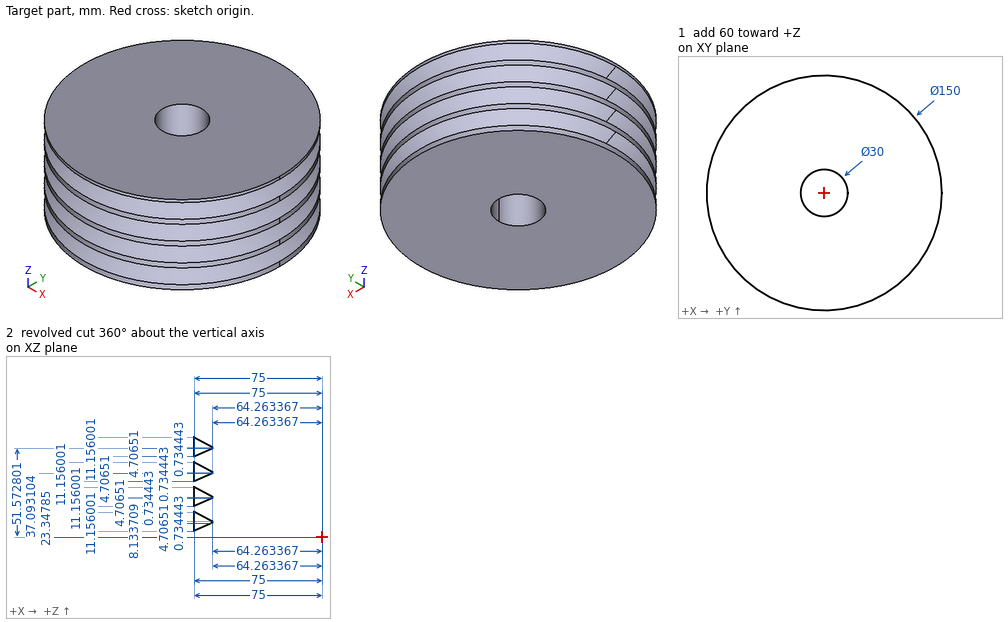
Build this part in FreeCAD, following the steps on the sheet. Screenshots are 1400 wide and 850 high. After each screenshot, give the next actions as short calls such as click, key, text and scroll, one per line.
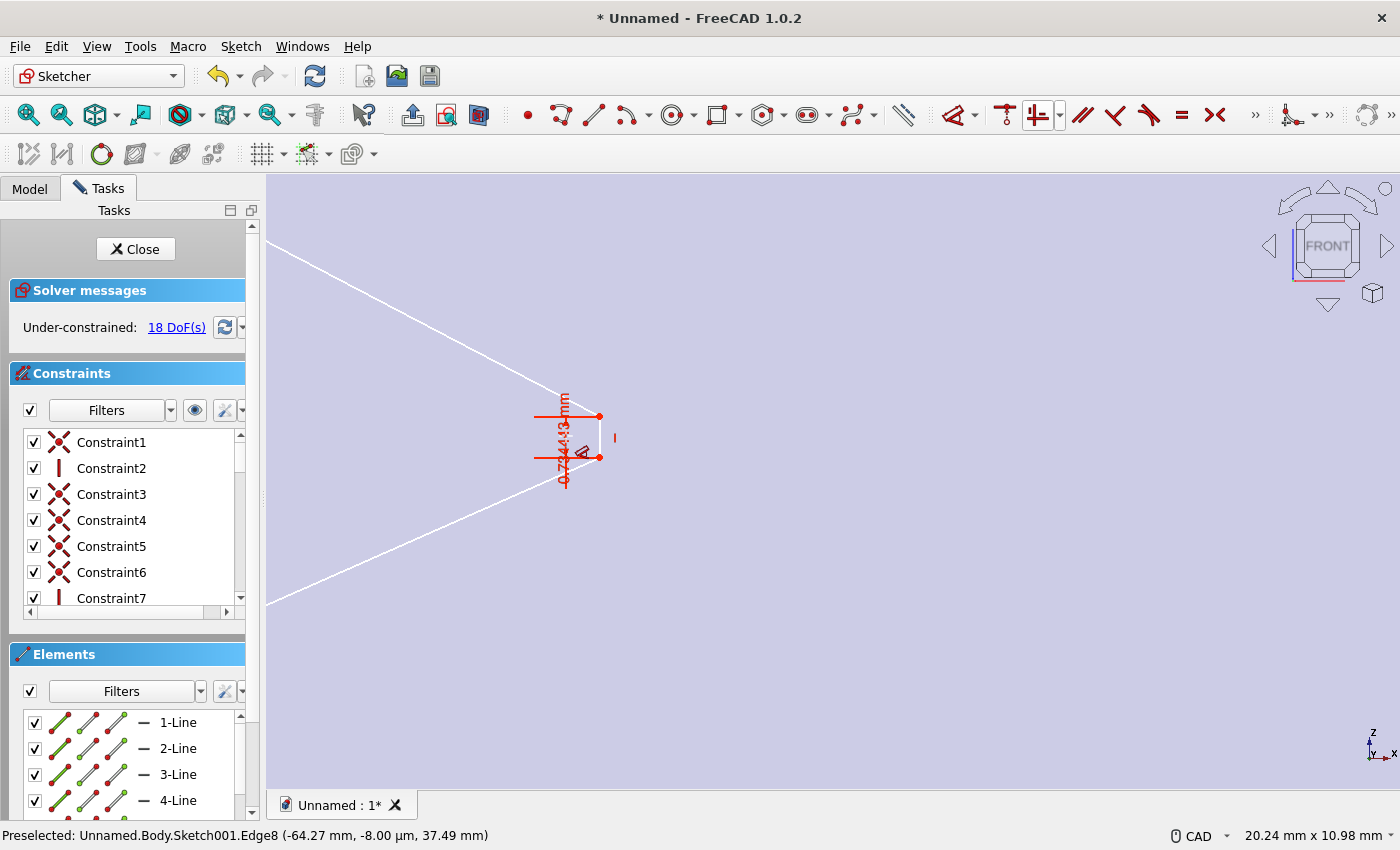
scroll(598, 429, down, 11)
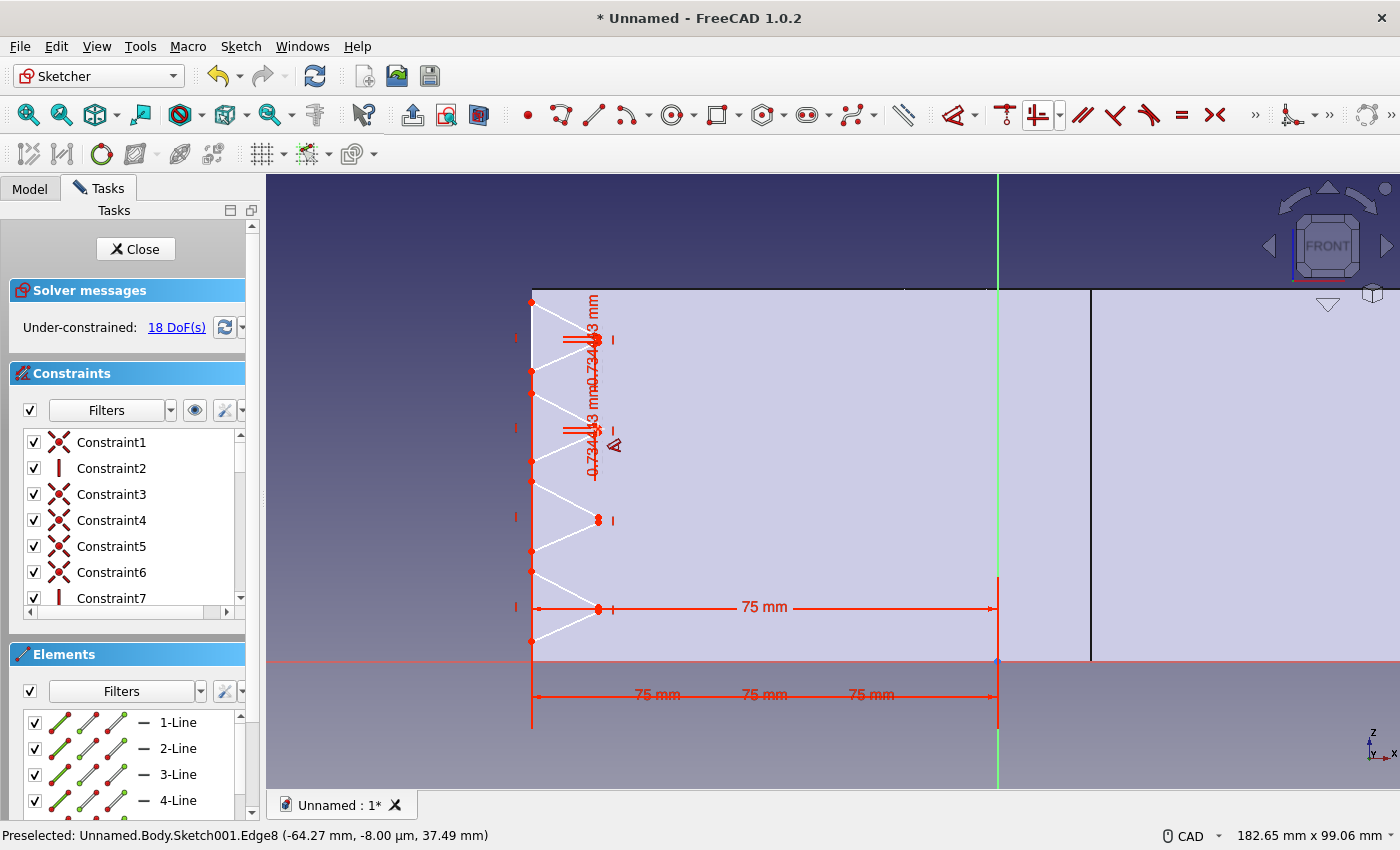
scroll(598, 519, up, 11)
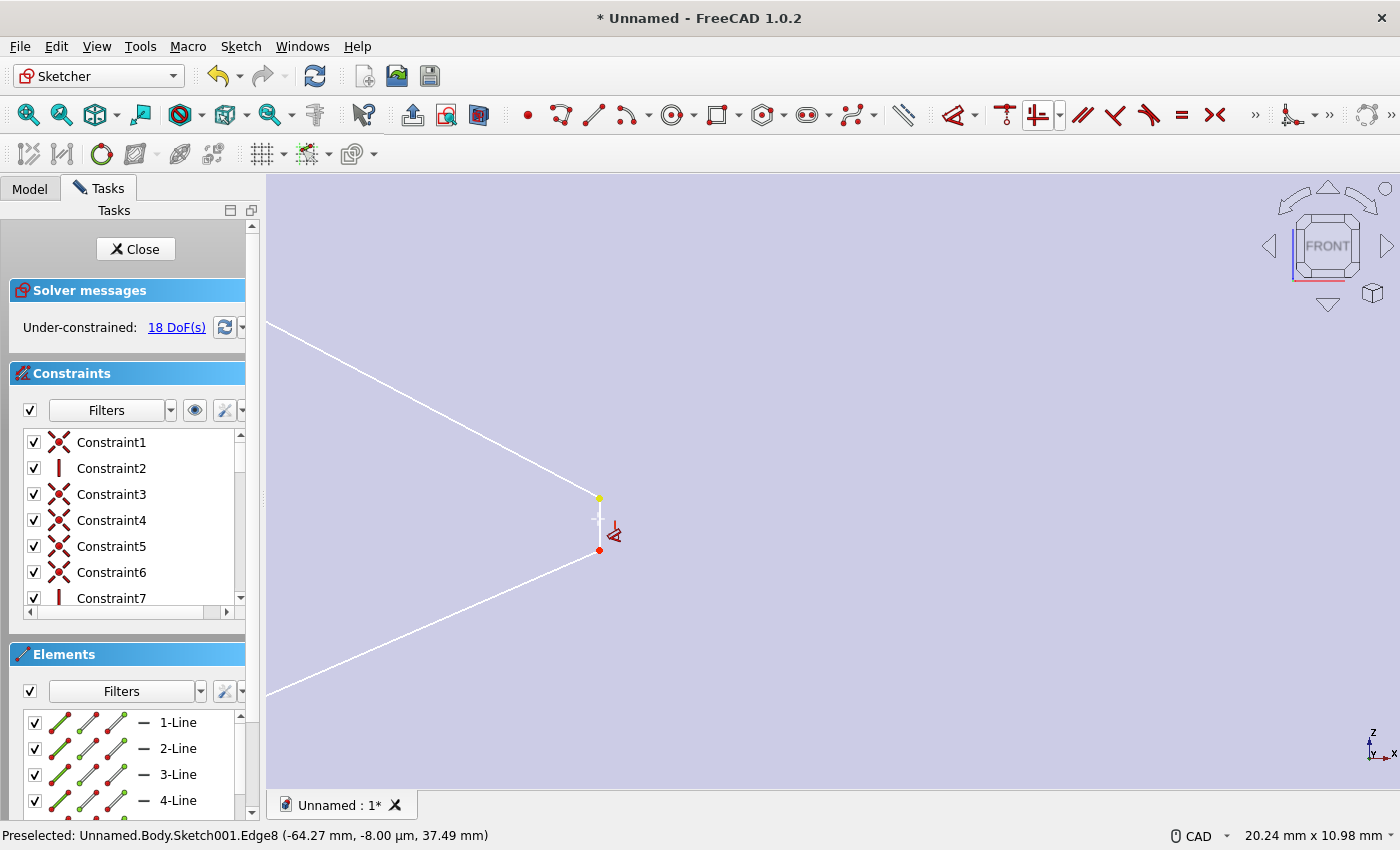
click(600, 514)
click(566, 524)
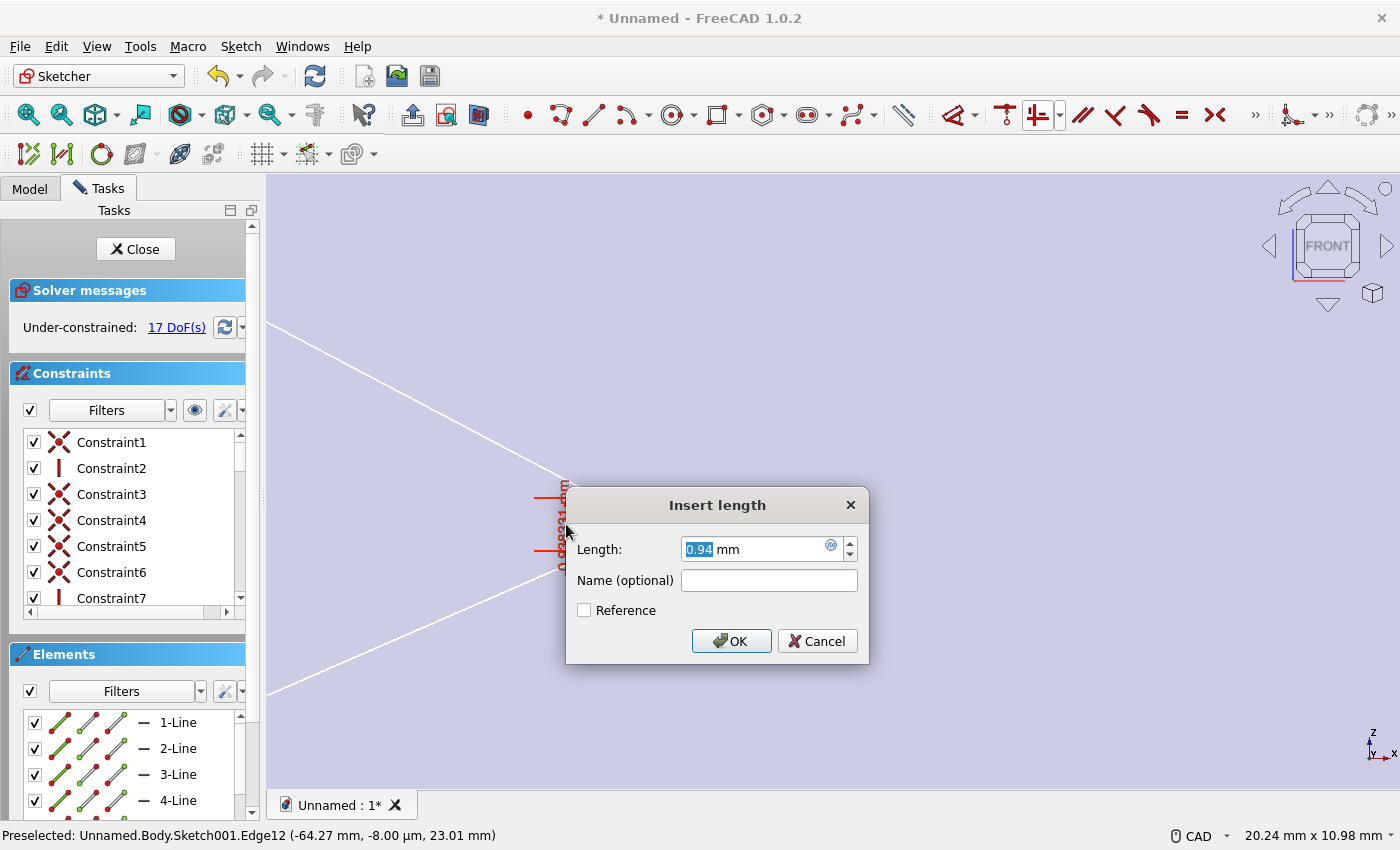
text(0.734443)
key(Return)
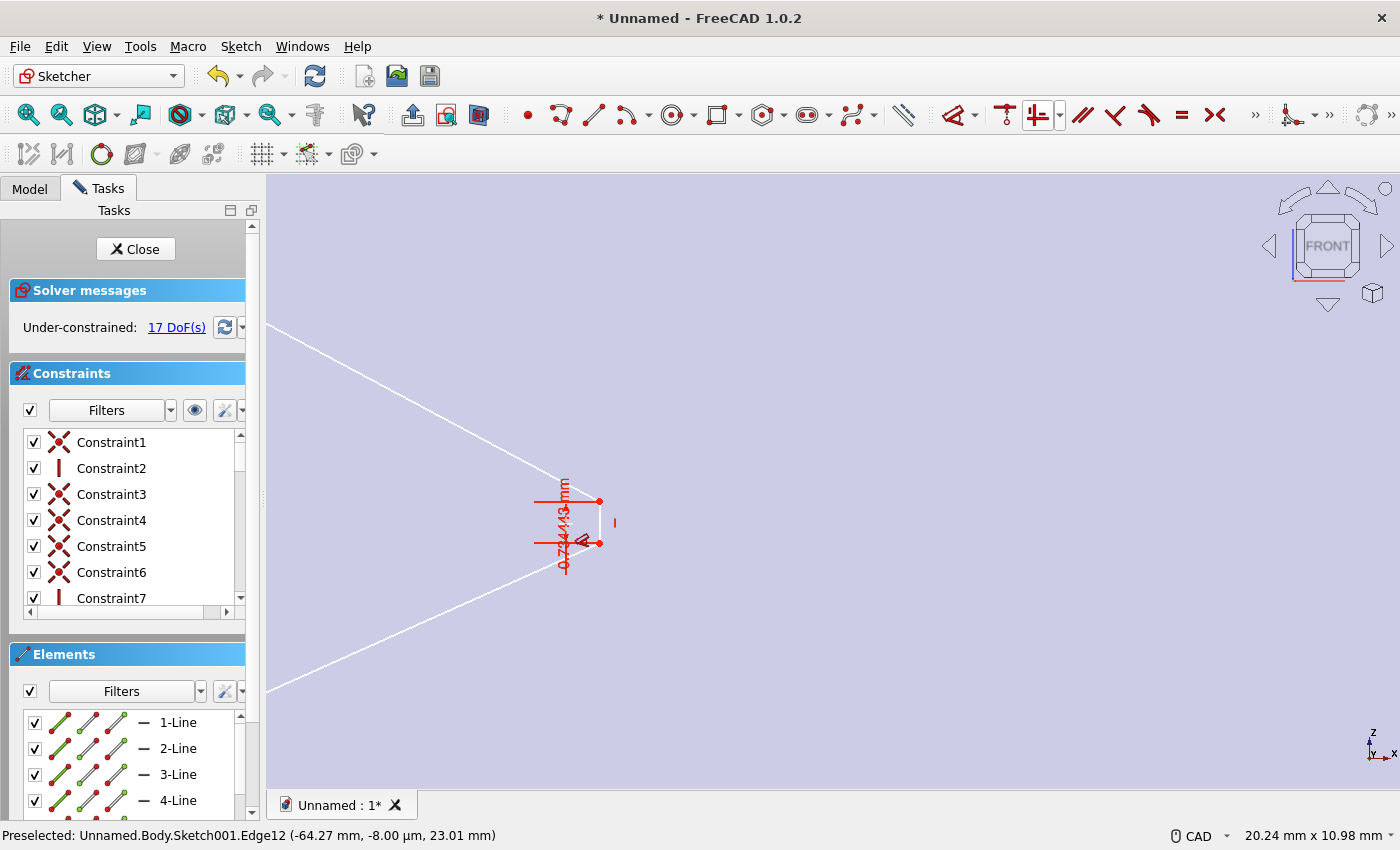
scroll(598, 519, down, 11)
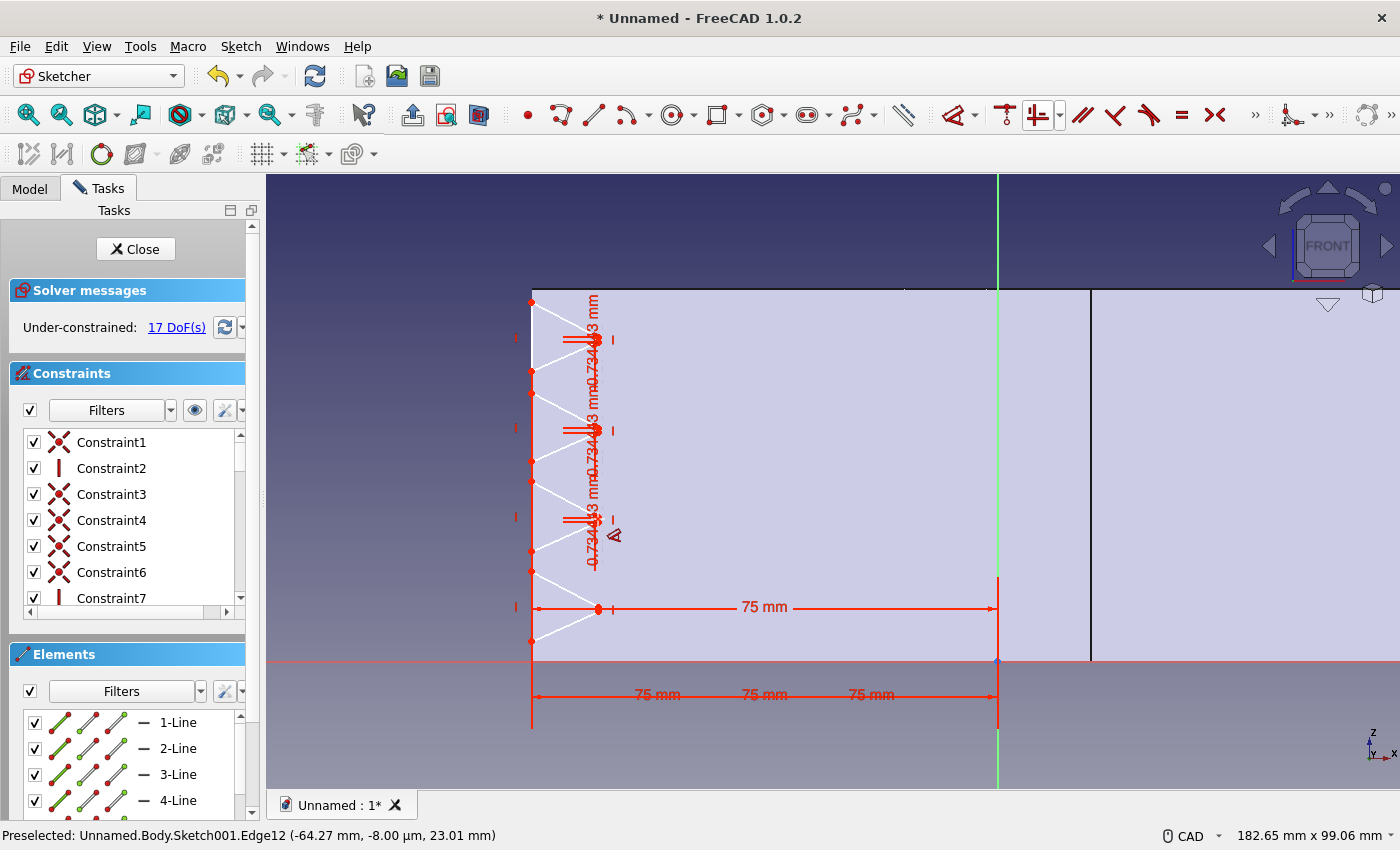
scroll(598, 609, up, 12)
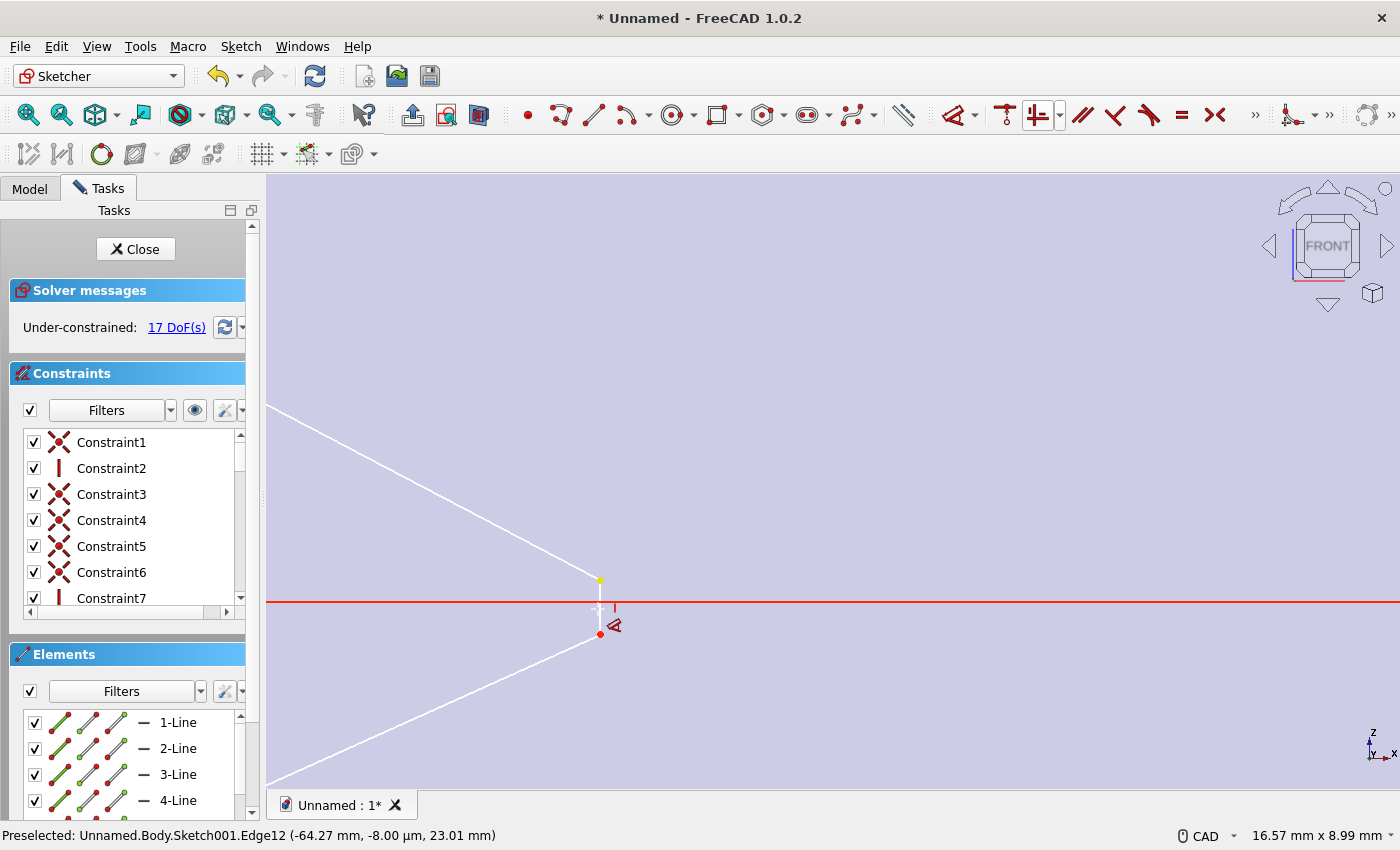
click(600, 597)
click(566, 608)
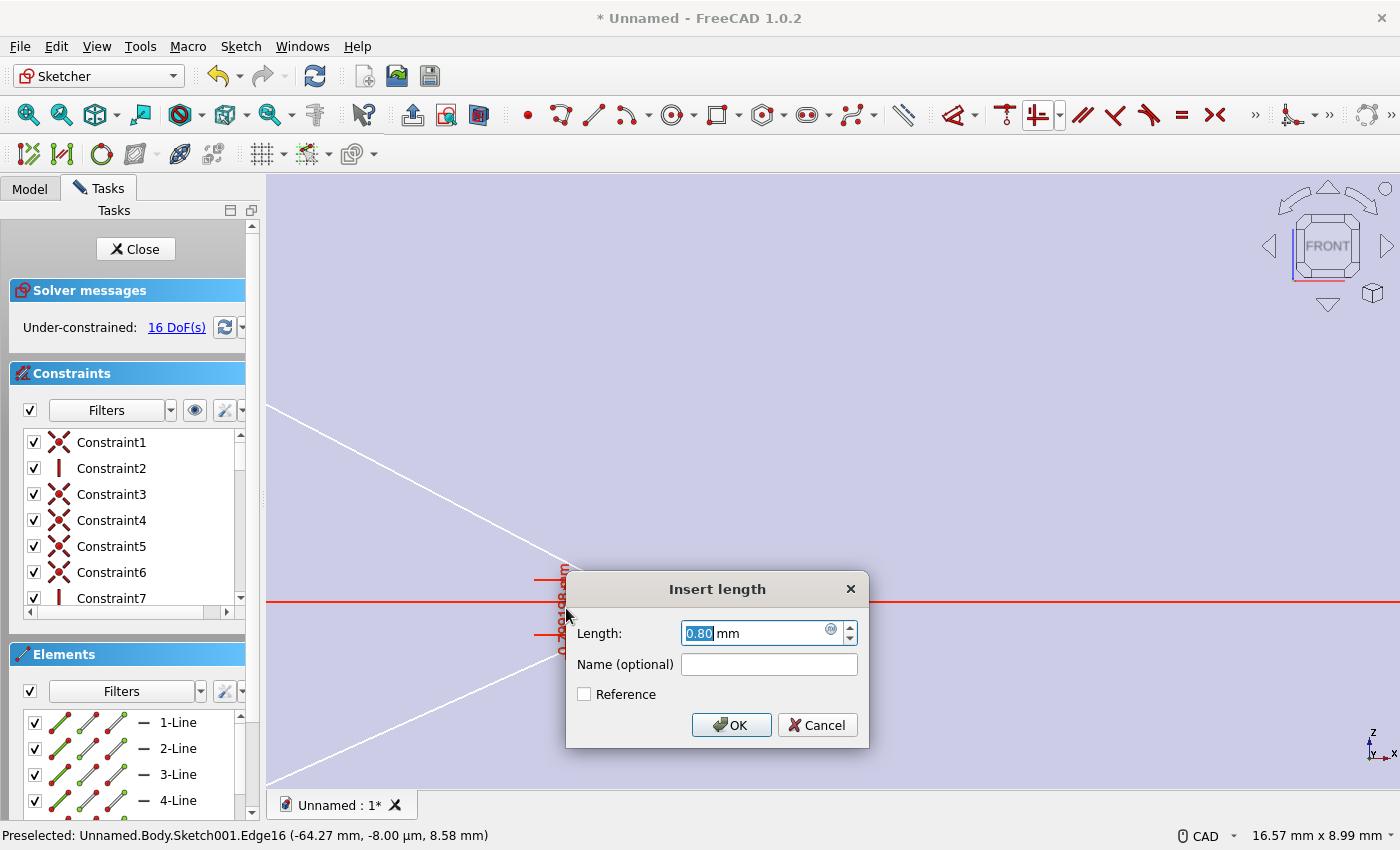
text(0.734443)
key(Return)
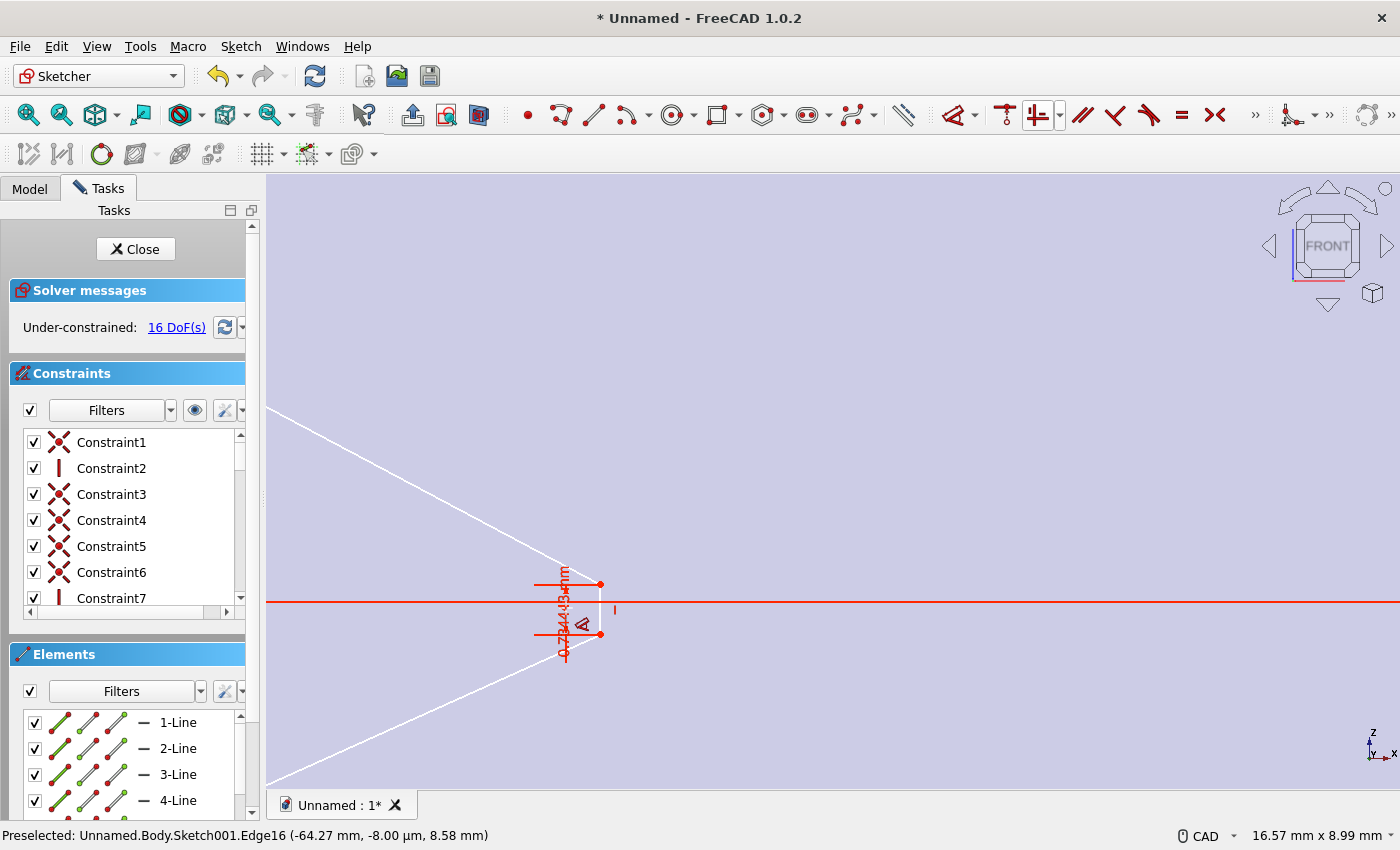
scroll(598, 609, down, 12)